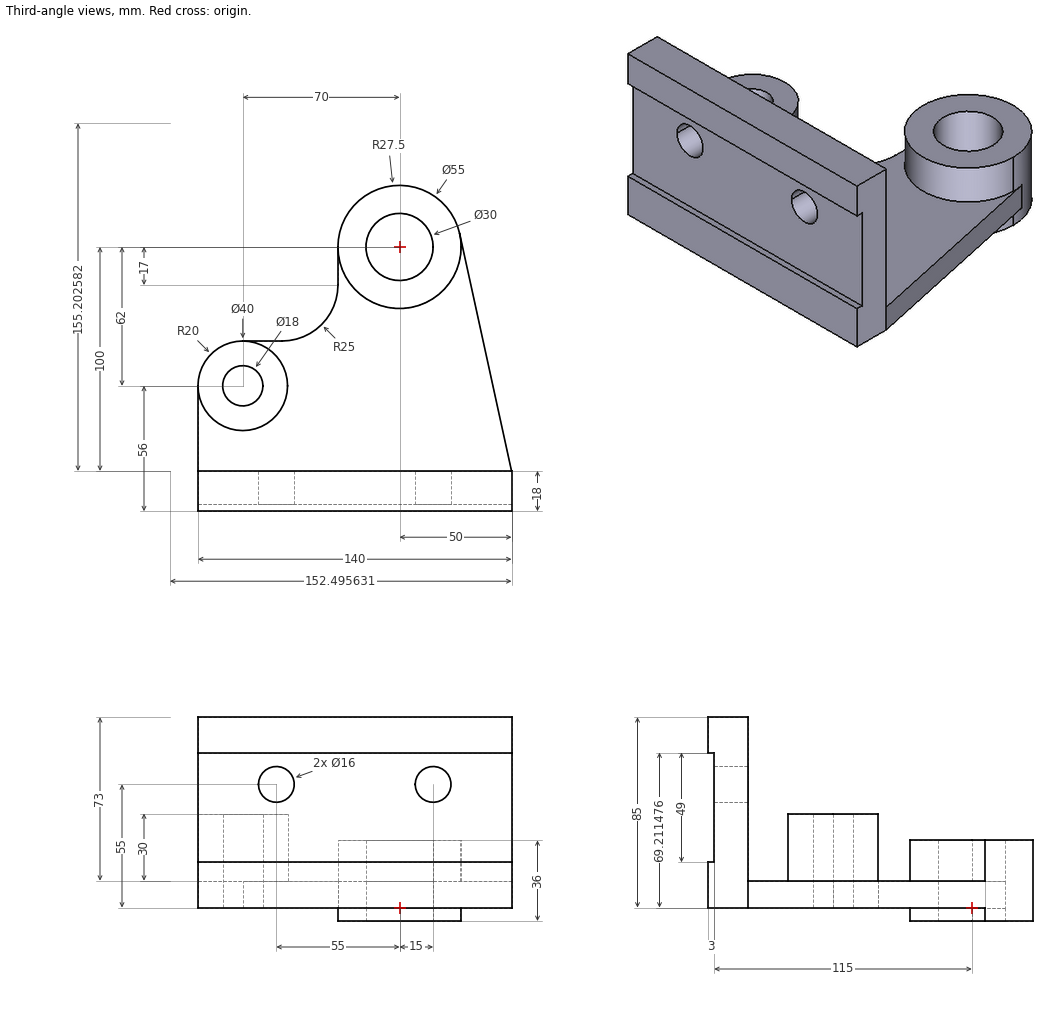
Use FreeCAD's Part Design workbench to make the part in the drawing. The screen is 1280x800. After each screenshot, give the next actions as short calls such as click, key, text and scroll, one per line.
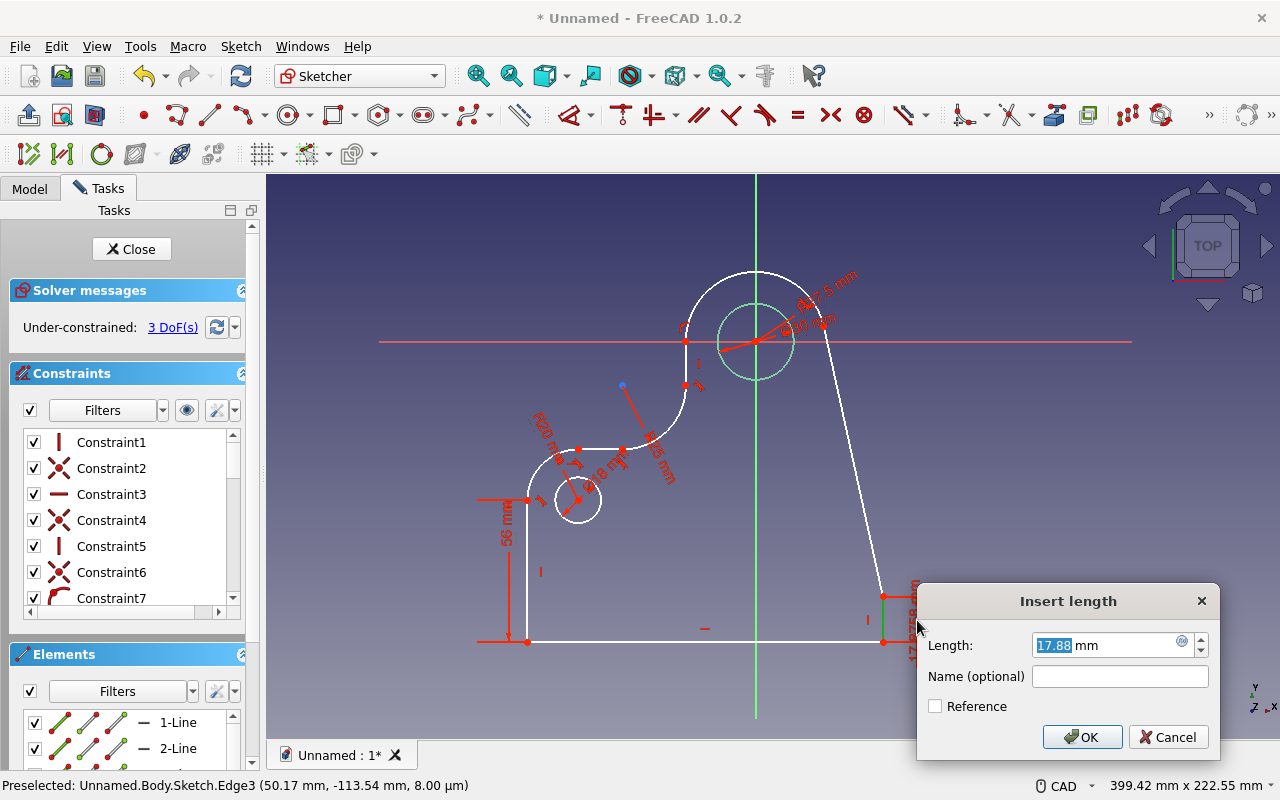
text(18)
key(Return)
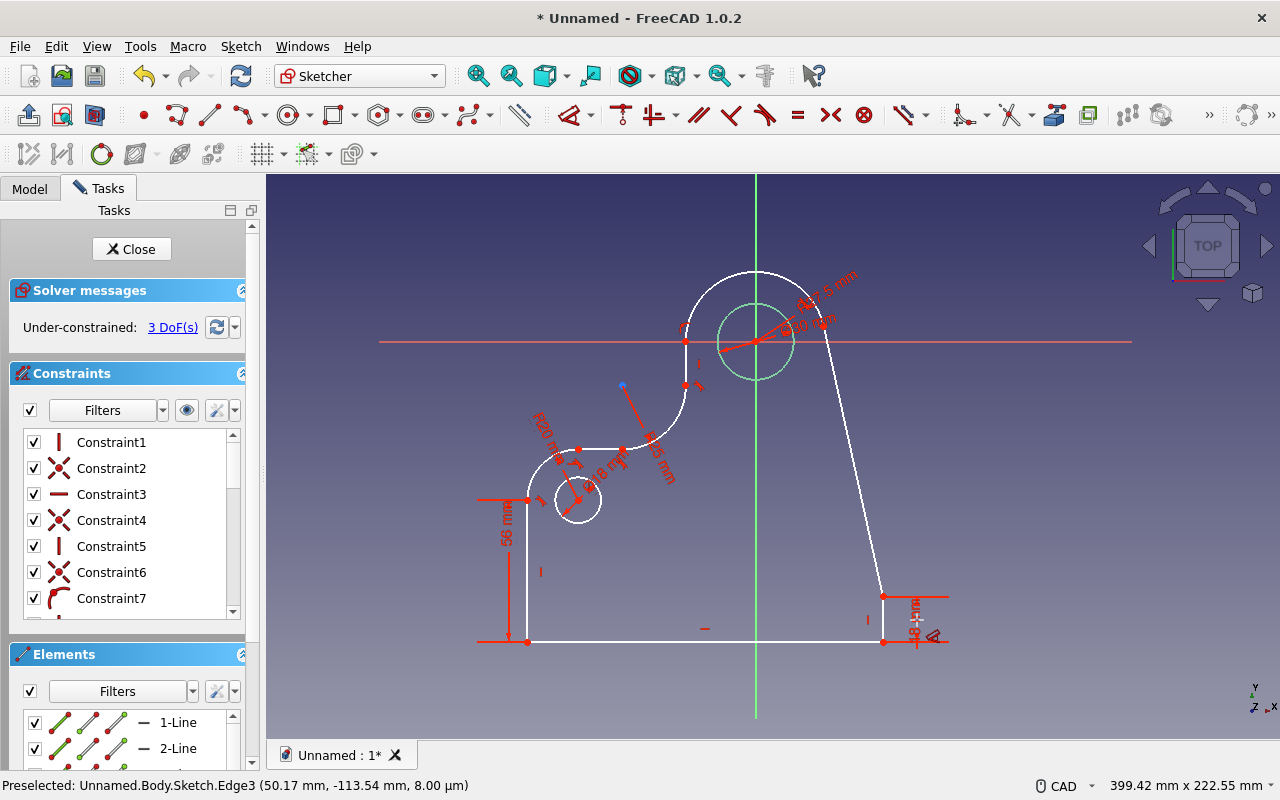
click(686, 355)
click(652, 364)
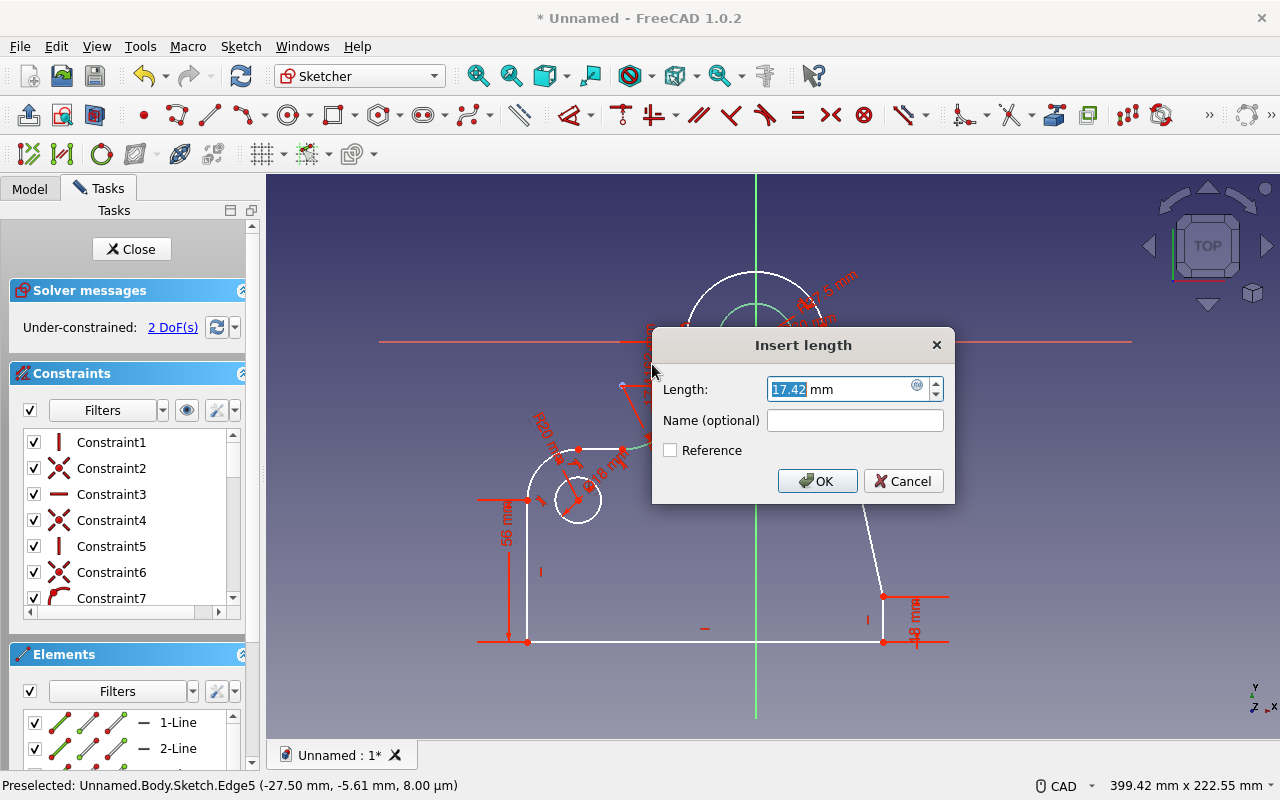
text(17)
key(Return)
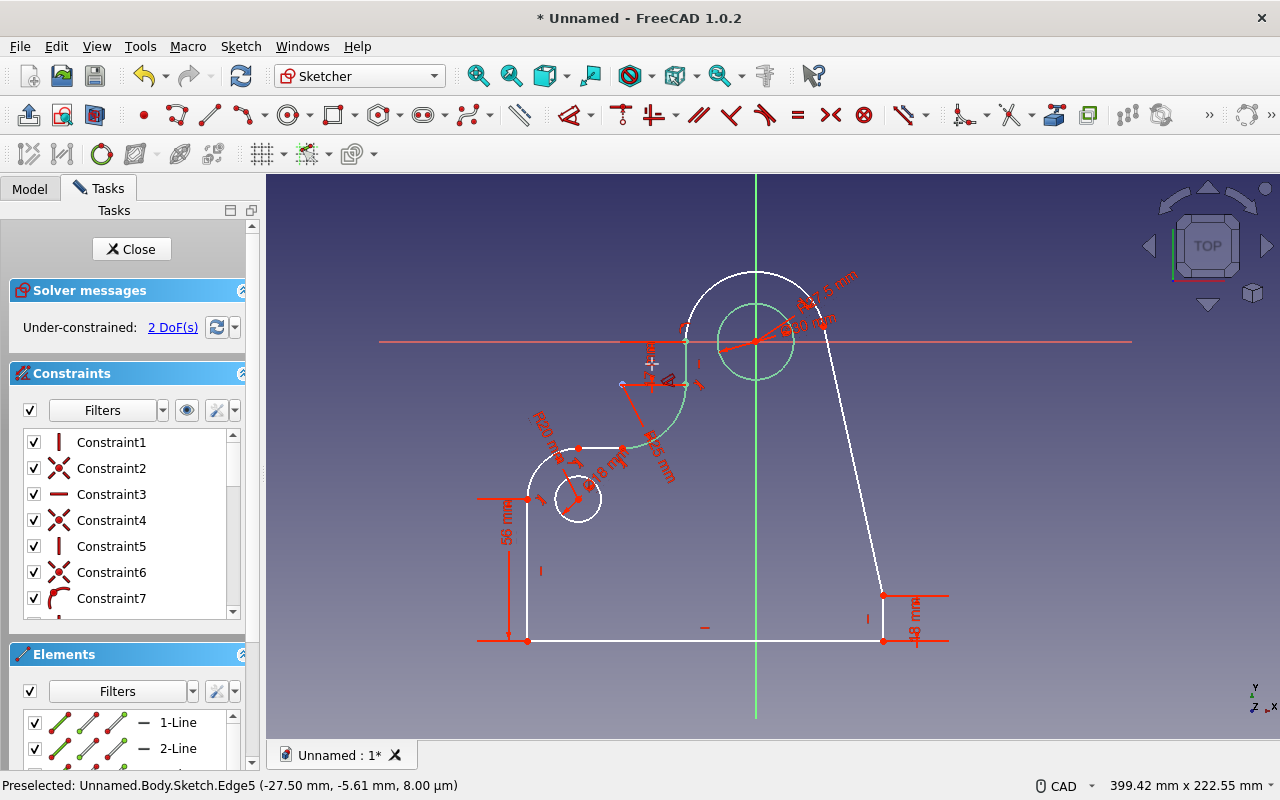
click(578, 499)
click(667, 308)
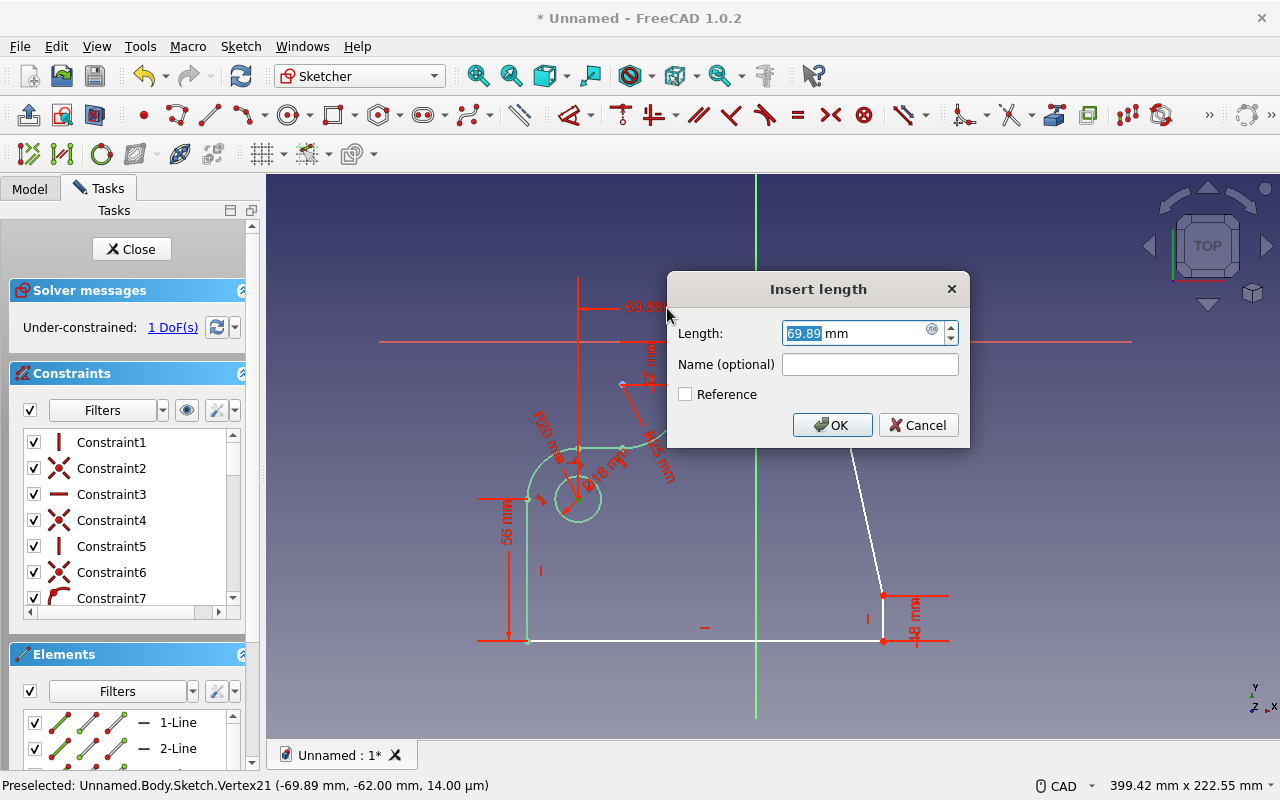
text(70)
key(Return)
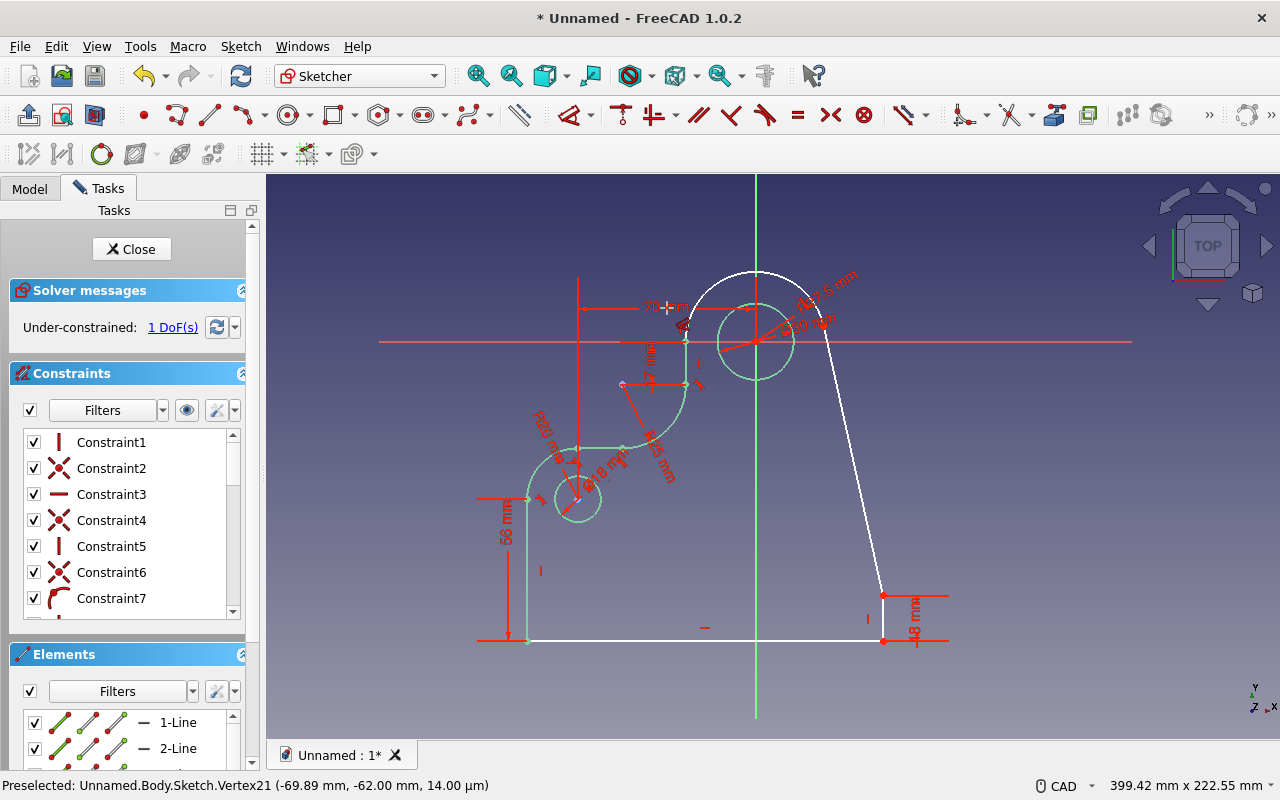
click(634, 641)
click(705, 675)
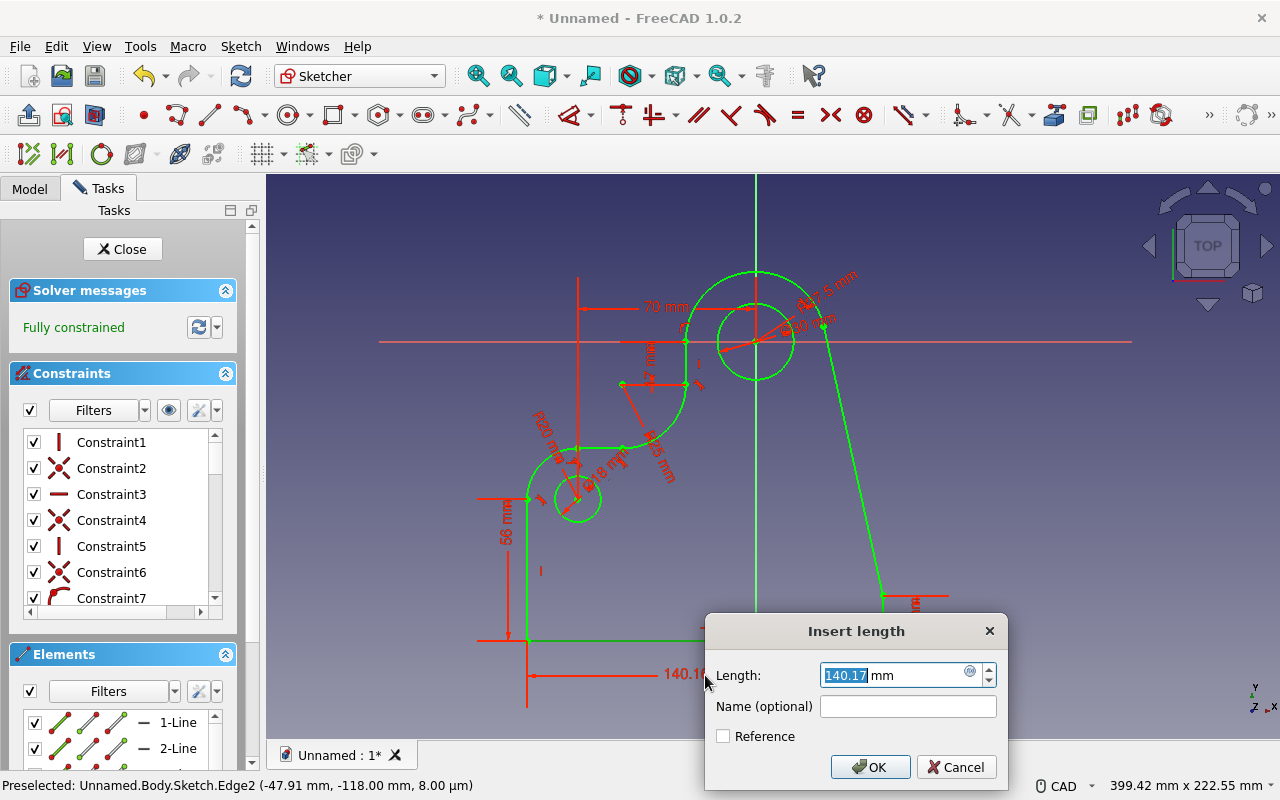
text(140)
key(Return)
key(Escape)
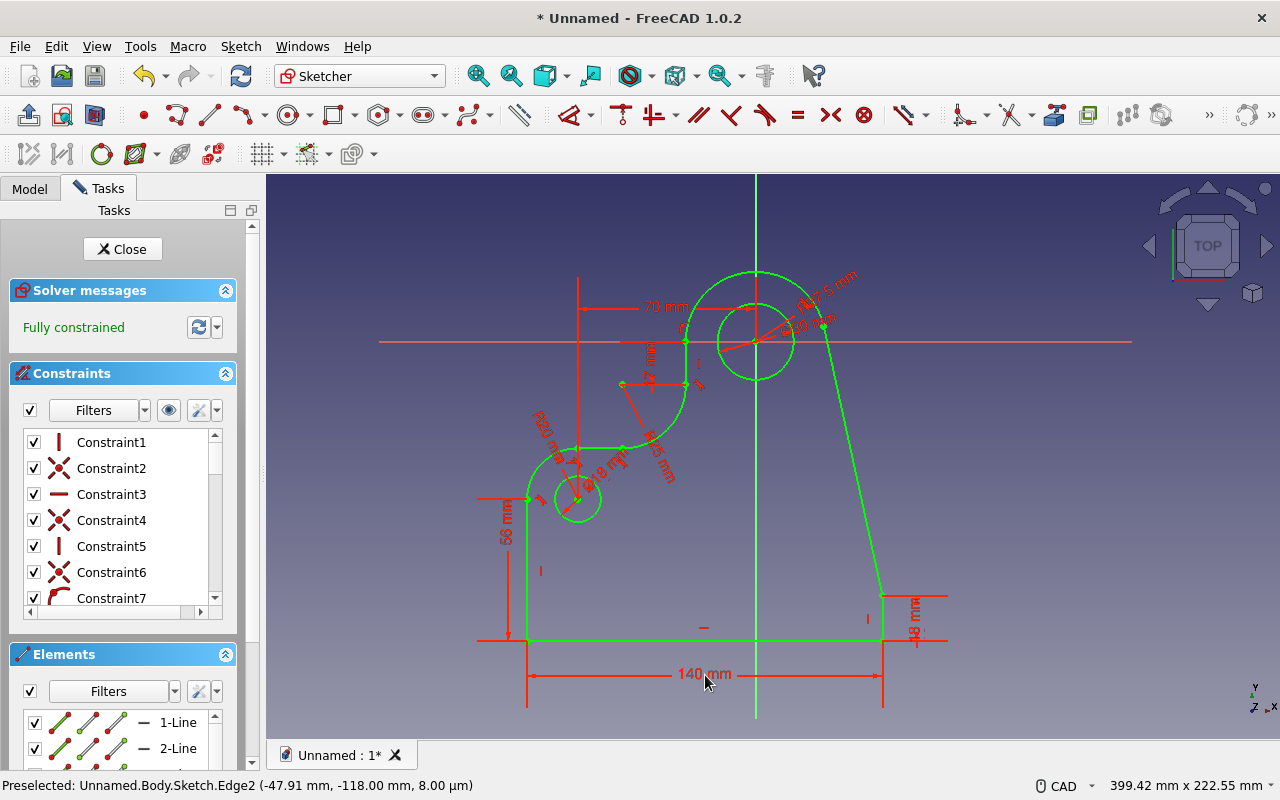
click(123, 249)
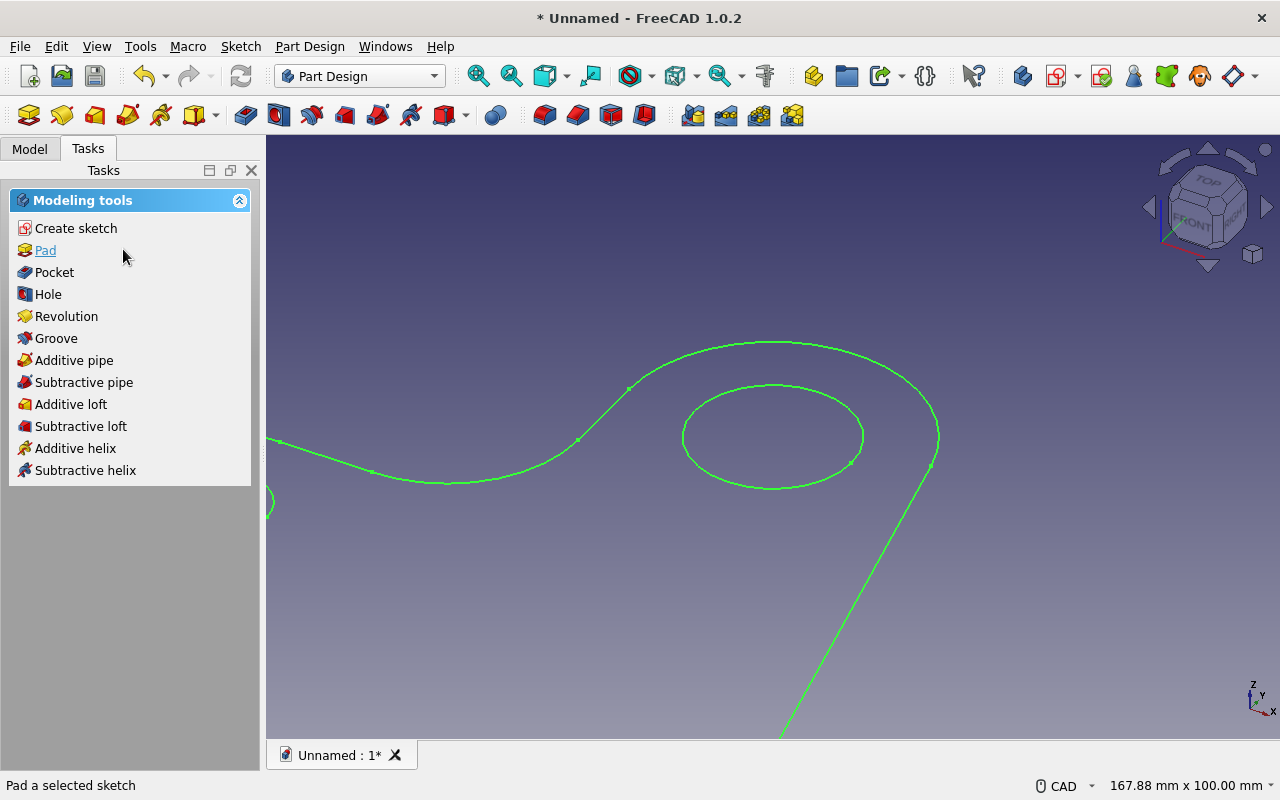
click(29, 116)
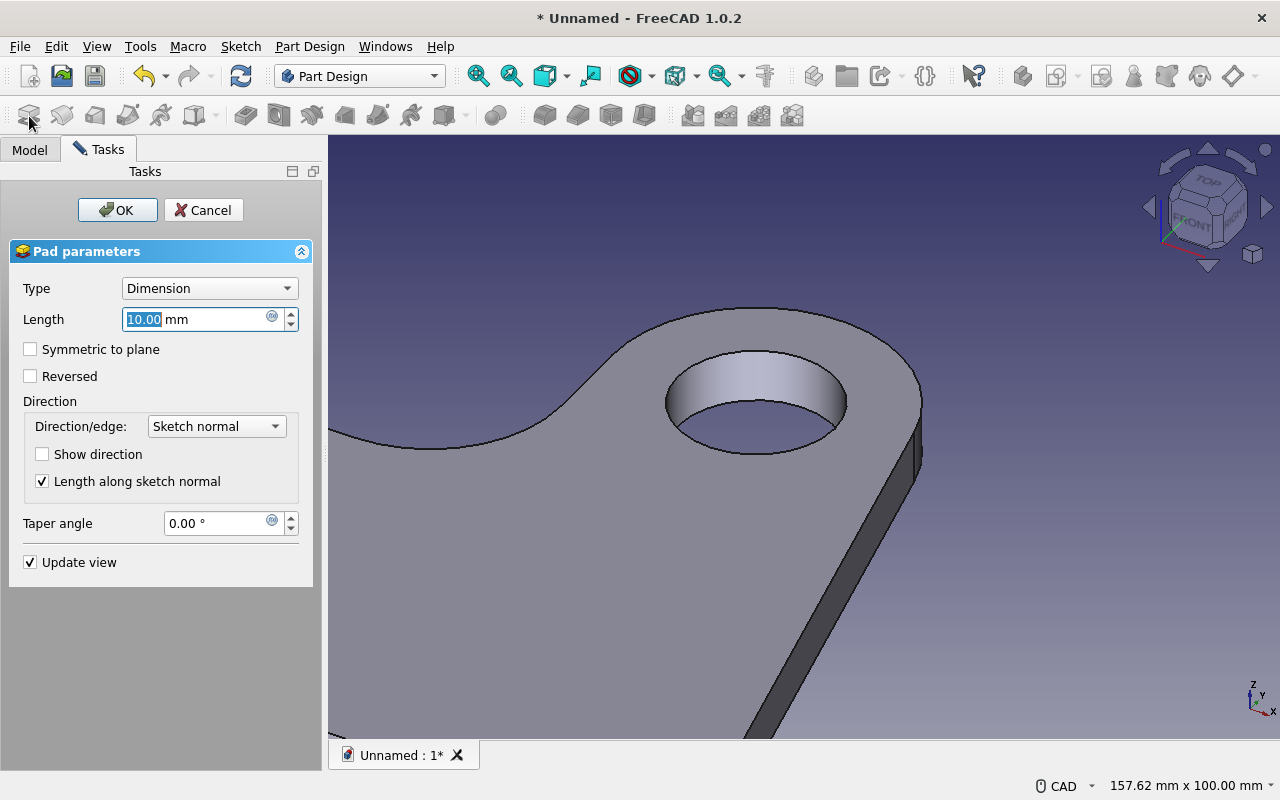
text(85)
key(Tab)